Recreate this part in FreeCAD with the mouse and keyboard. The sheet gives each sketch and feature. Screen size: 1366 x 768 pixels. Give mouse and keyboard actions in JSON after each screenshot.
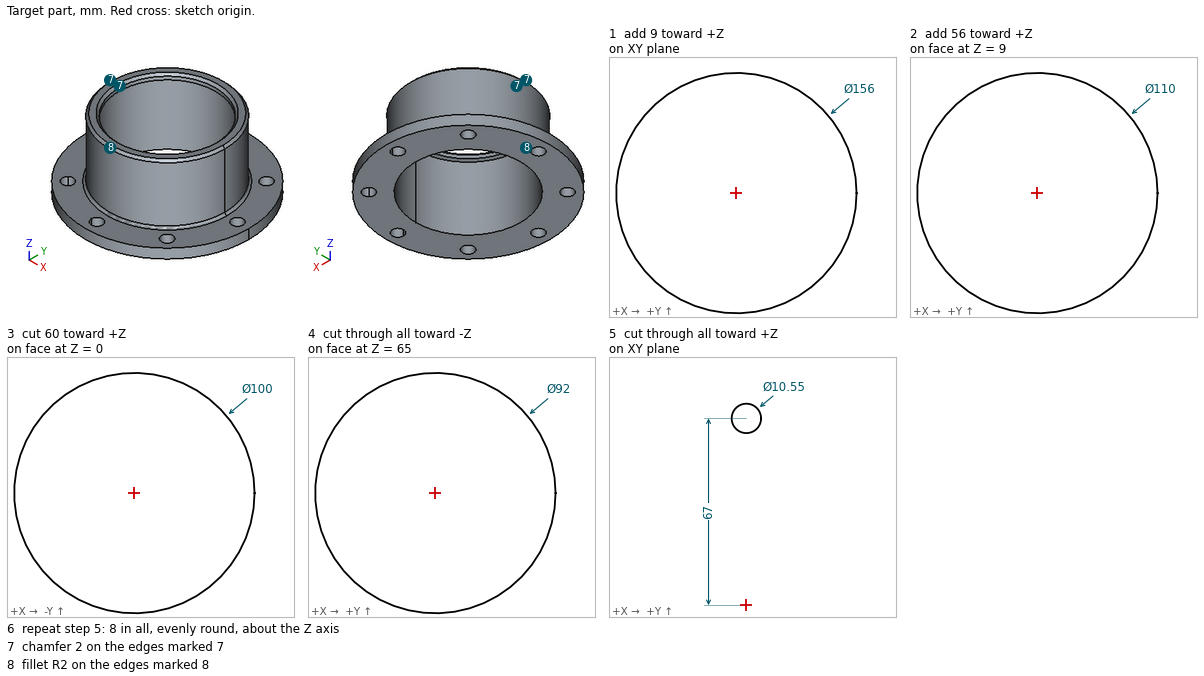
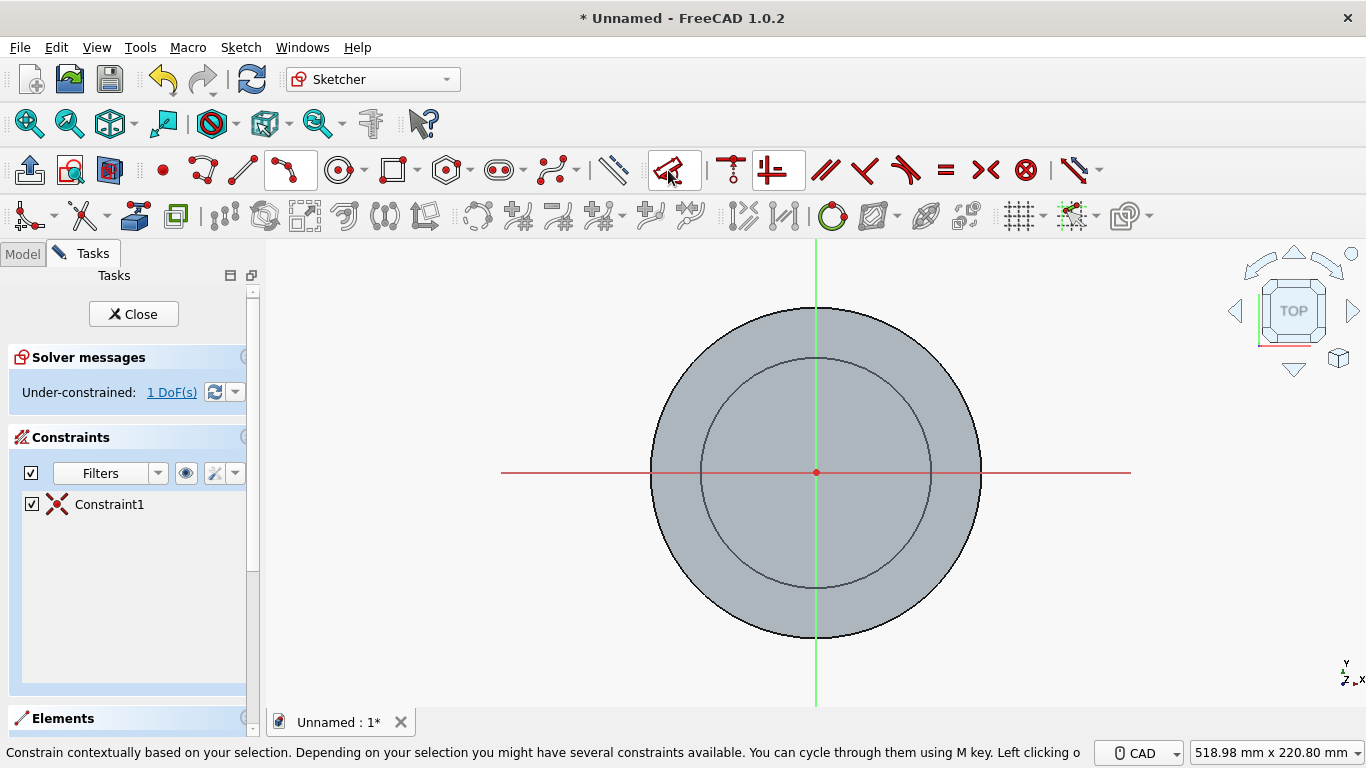
{"action": "left_click", "coordinate": [897, 391]}
{"action": "left_click", "coordinate": [919, 368]}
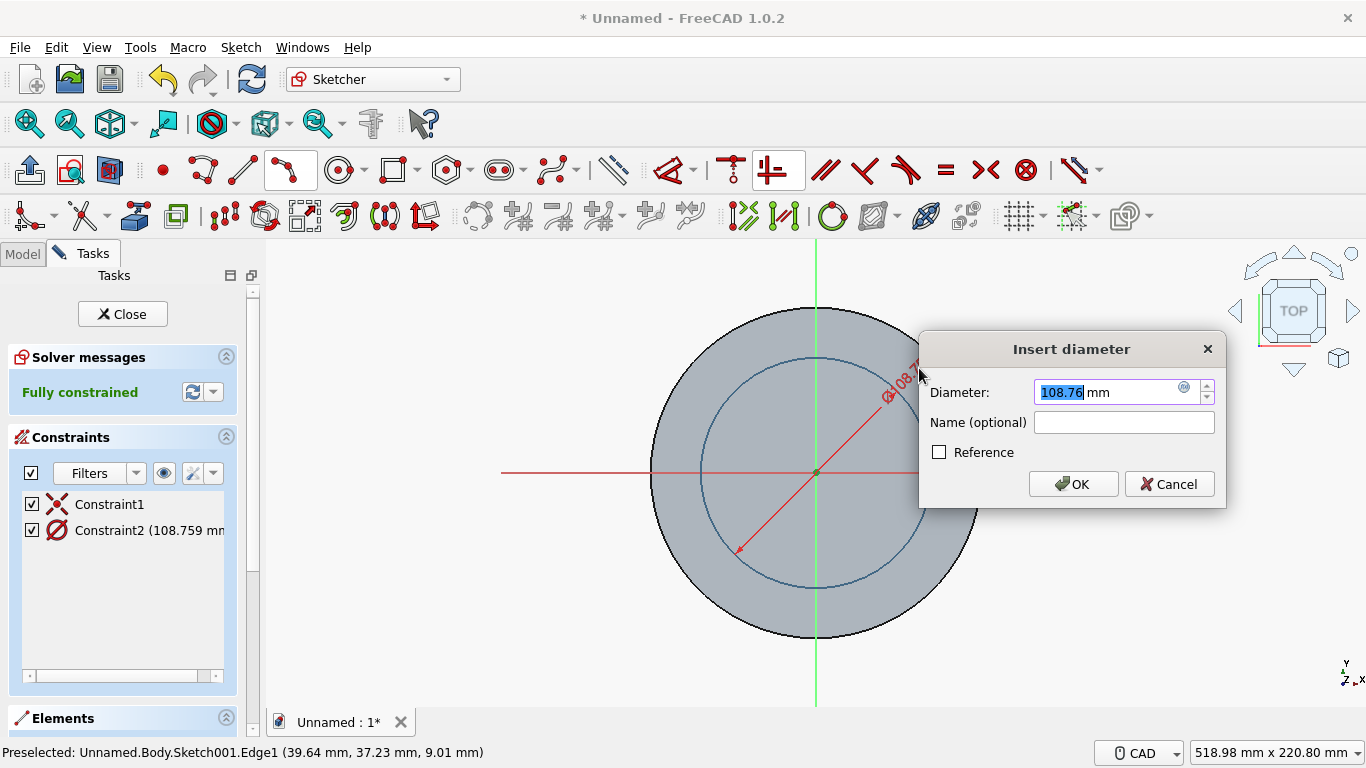
{"action": "type", "text": "110"}
{"action": "key", "text": "Return"}
{"action": "key", "text": "Escape"}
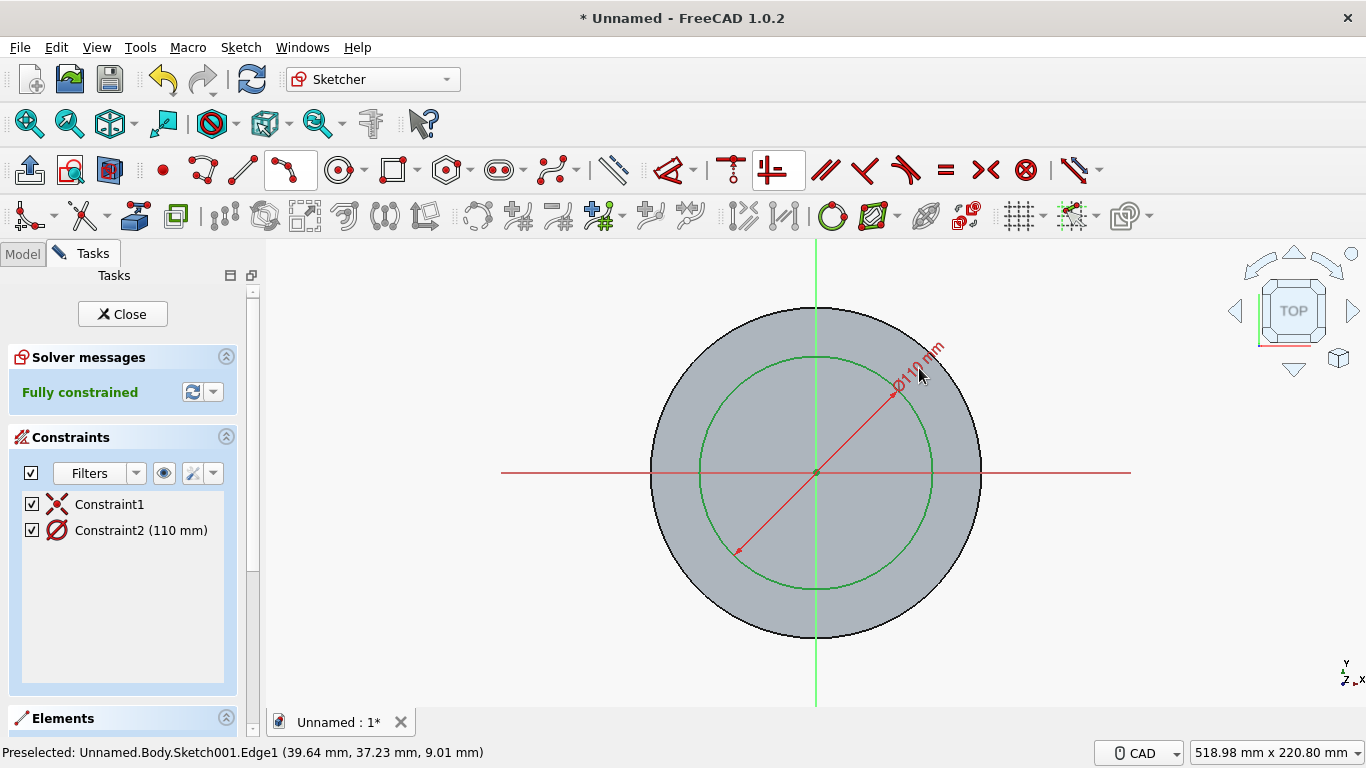
{"action": "left_click", "coordinate": [123, 314]}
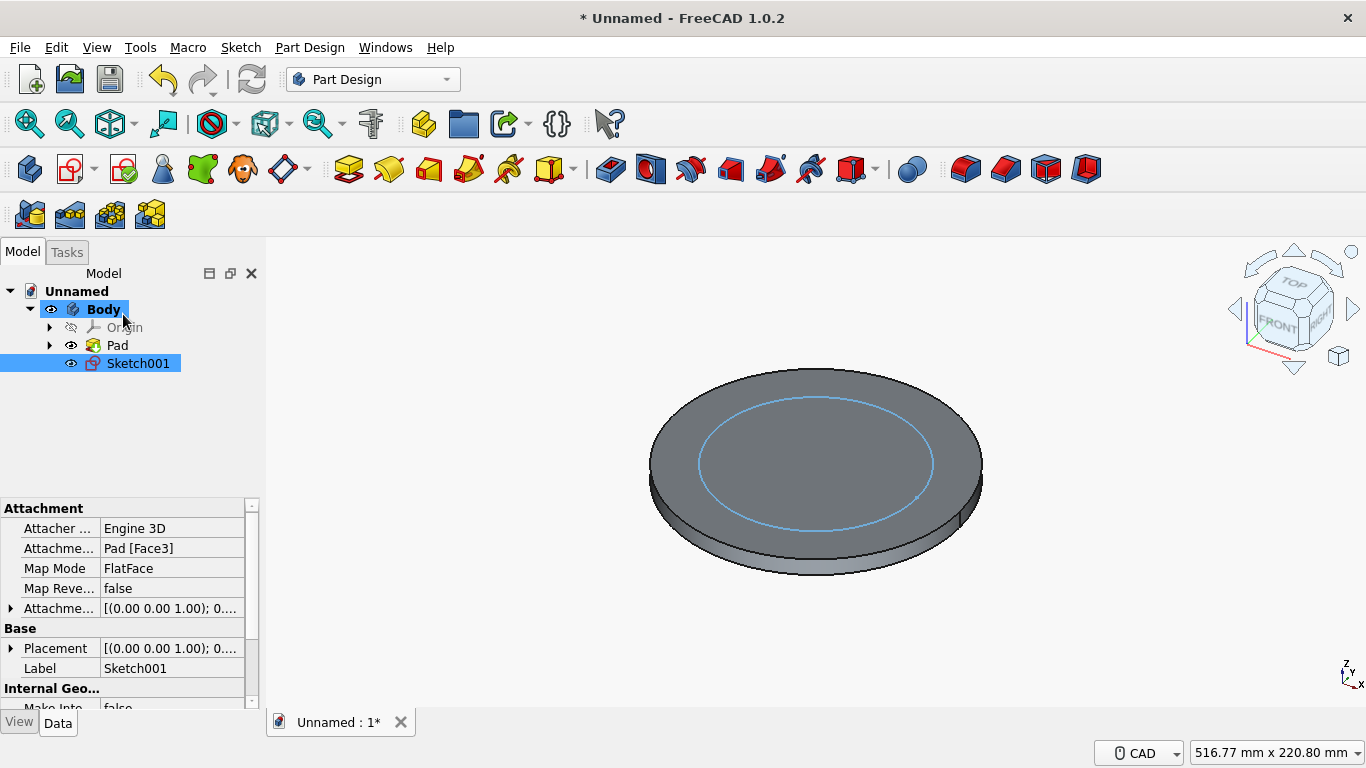
{"action": "left_click", "coordinate": [350, 170]}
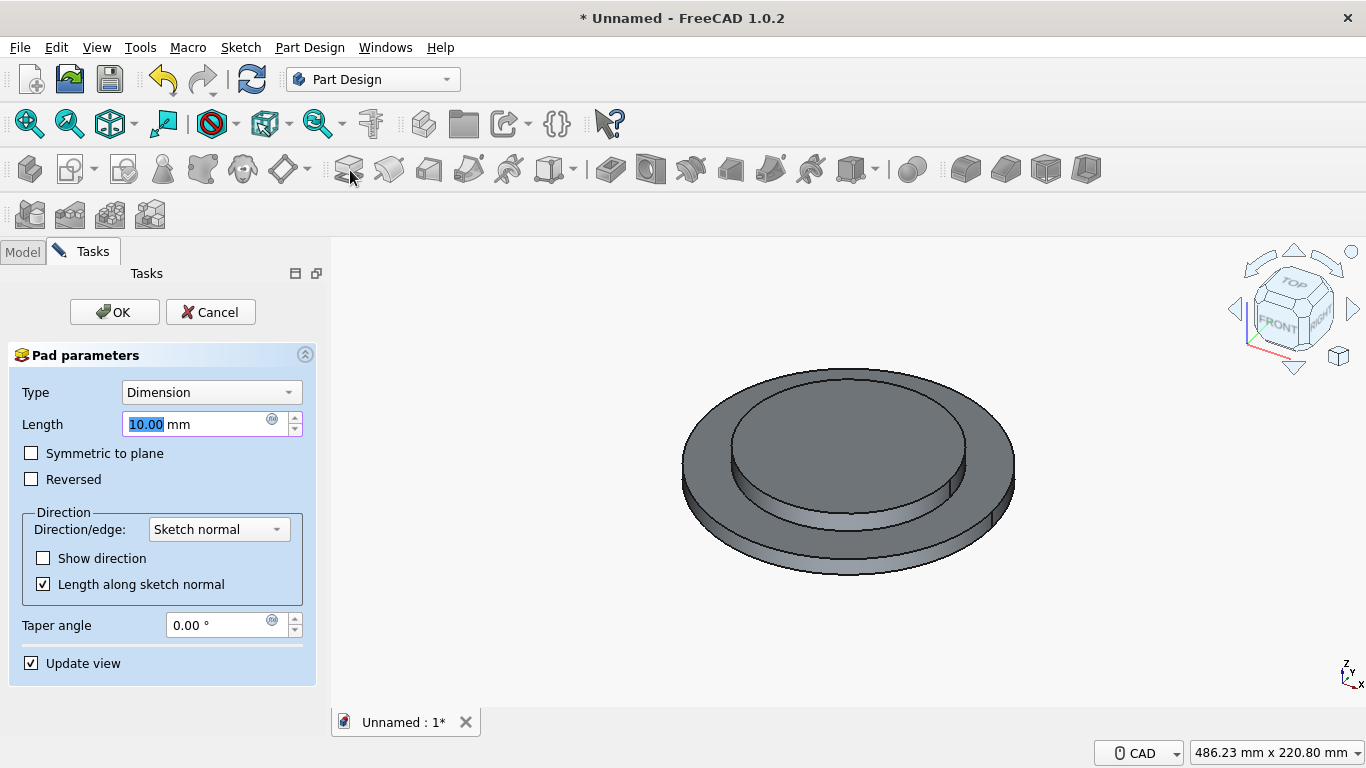
{"action": "type", "text": "56"}
{"action": "key", "text": "Tab"}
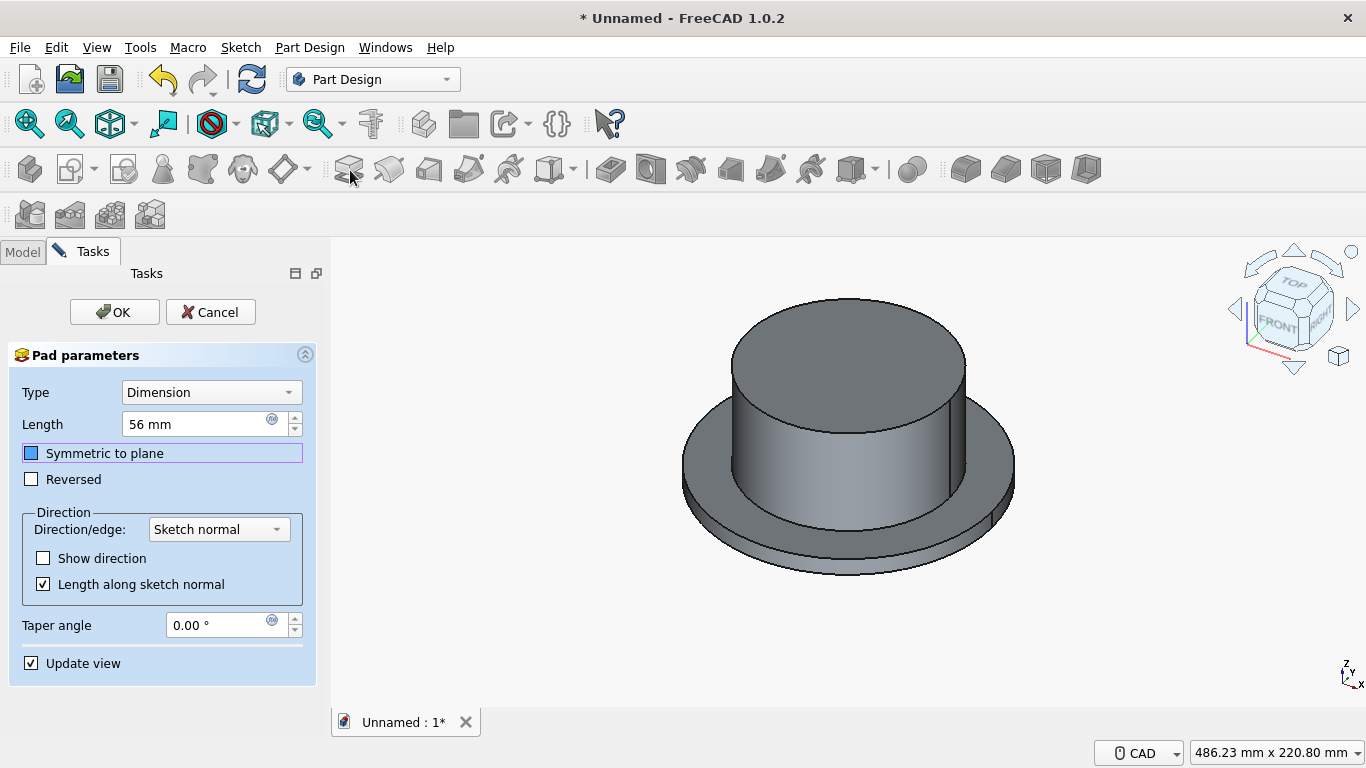
{"action": "left_click", "coordinate": [115, 312]}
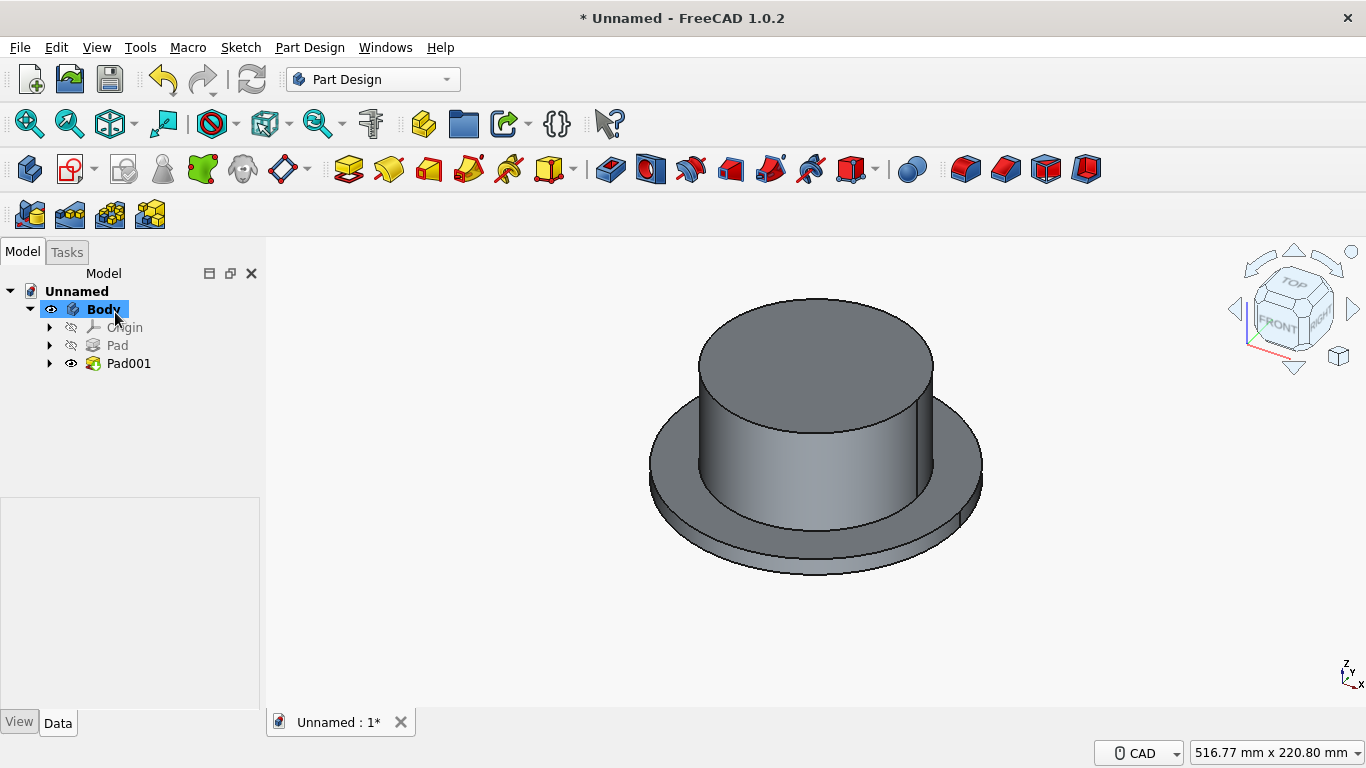
{"action": "left_click", "coordinate": [30, 124]}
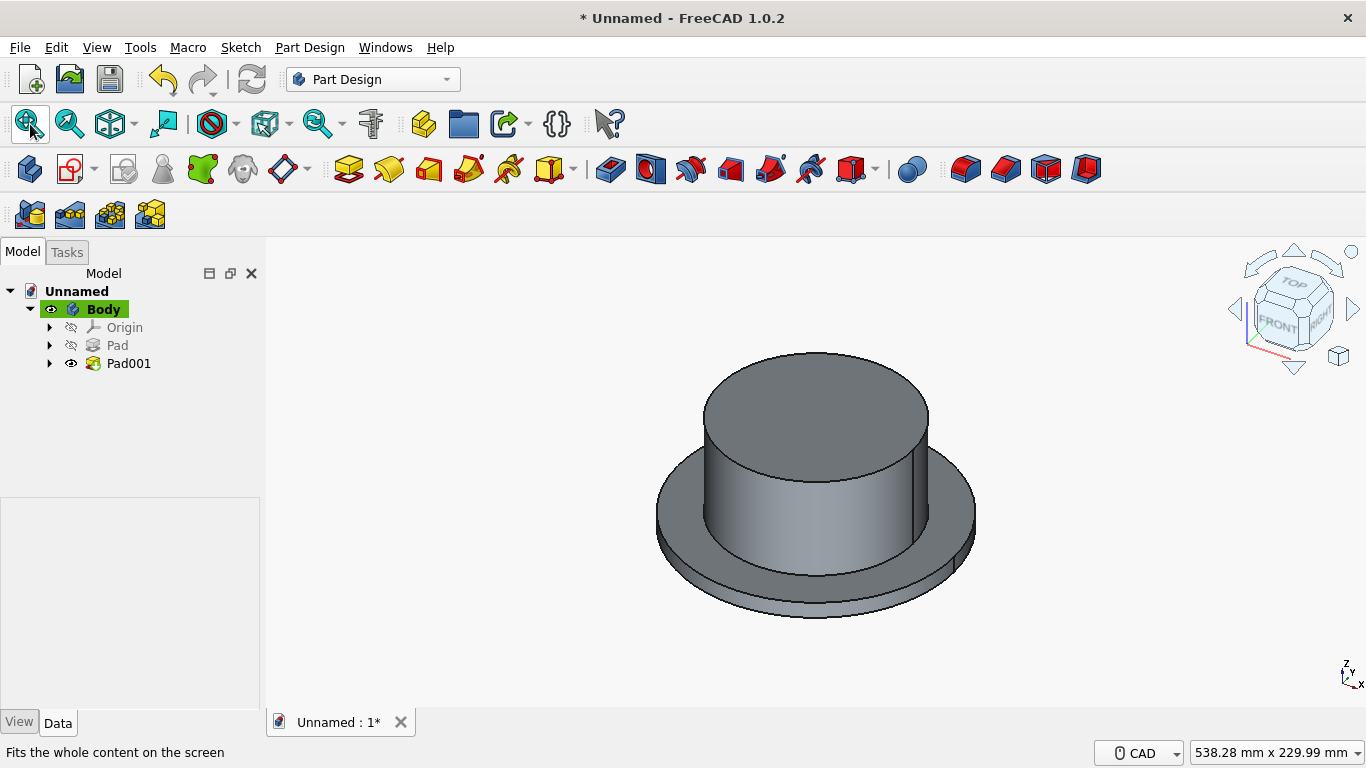
{"action": "key", "text": "5"}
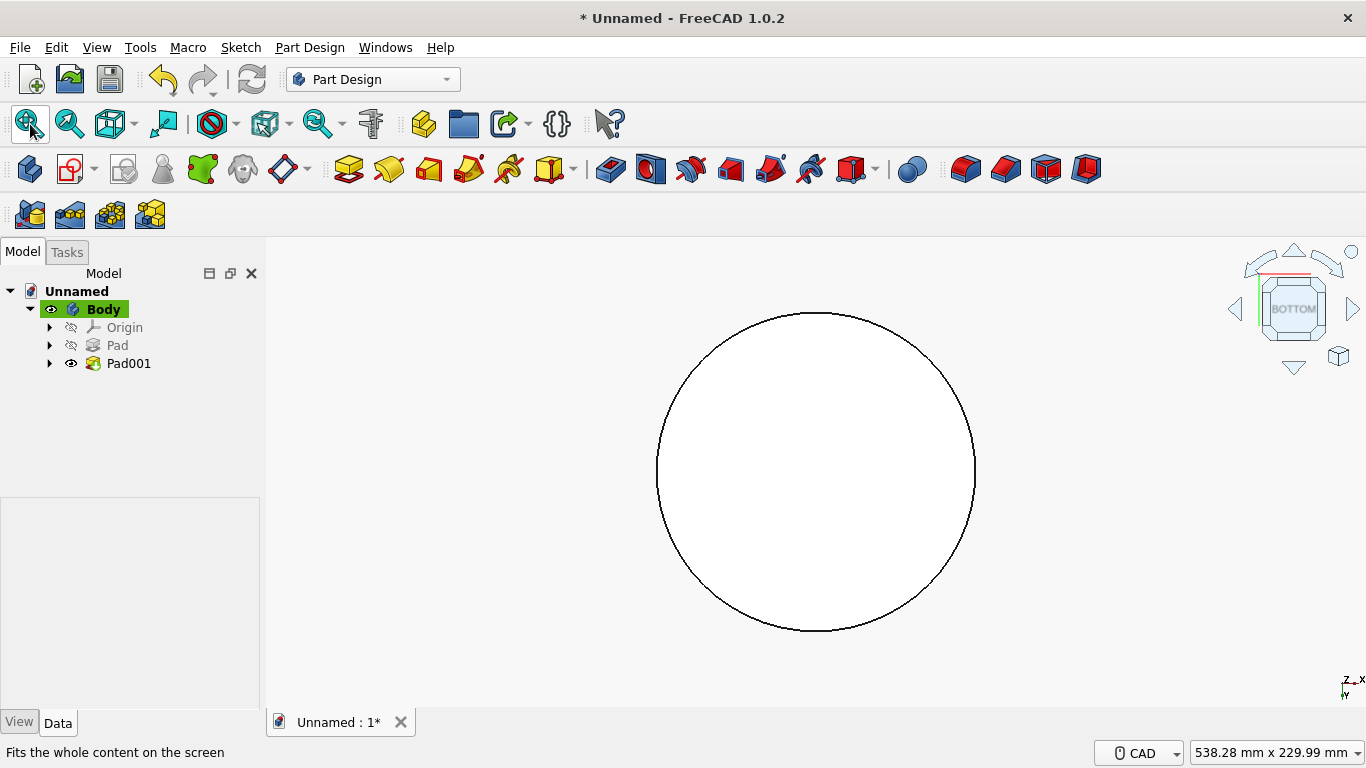
{"action": "left_click", "coordinate": [816, 471]}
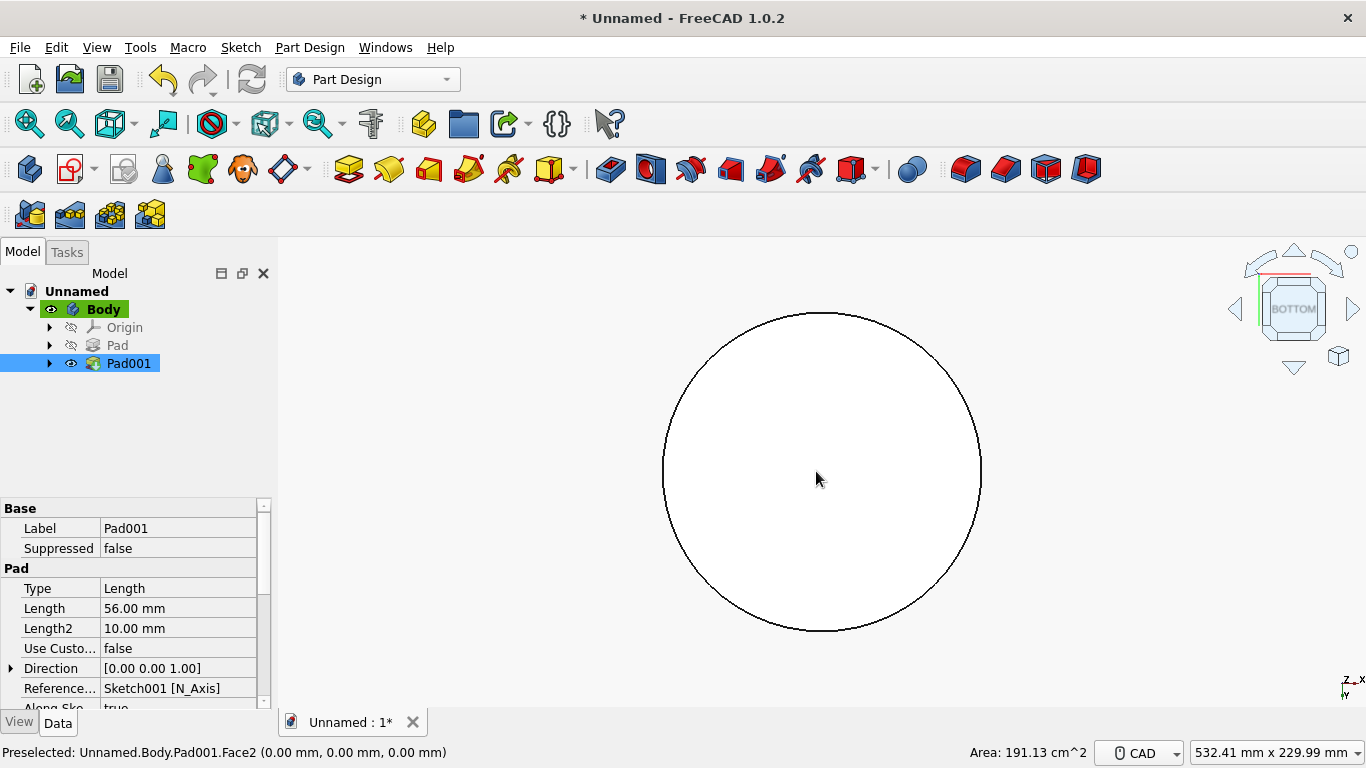
{"action": "left_click", "coordinate": [70, 170]}